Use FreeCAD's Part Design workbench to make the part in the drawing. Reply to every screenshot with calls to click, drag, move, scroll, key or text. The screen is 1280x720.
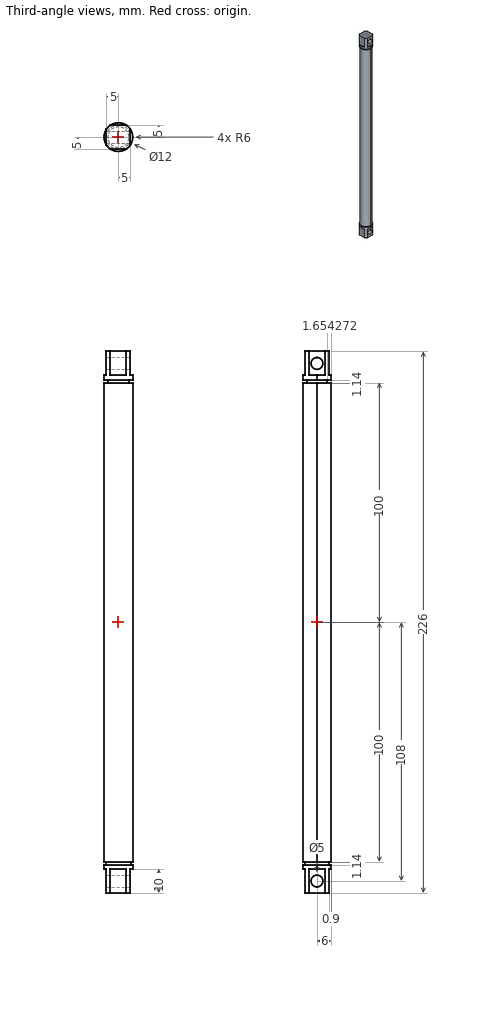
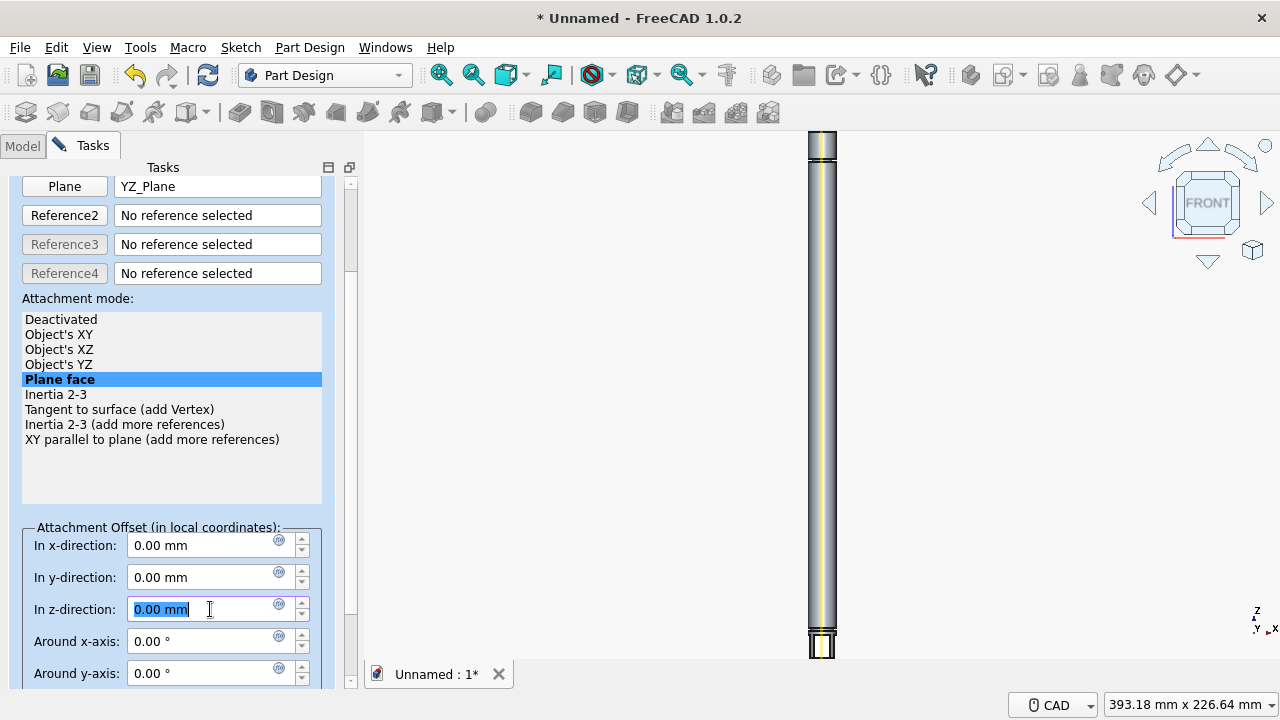
text(-5)
key(Tab)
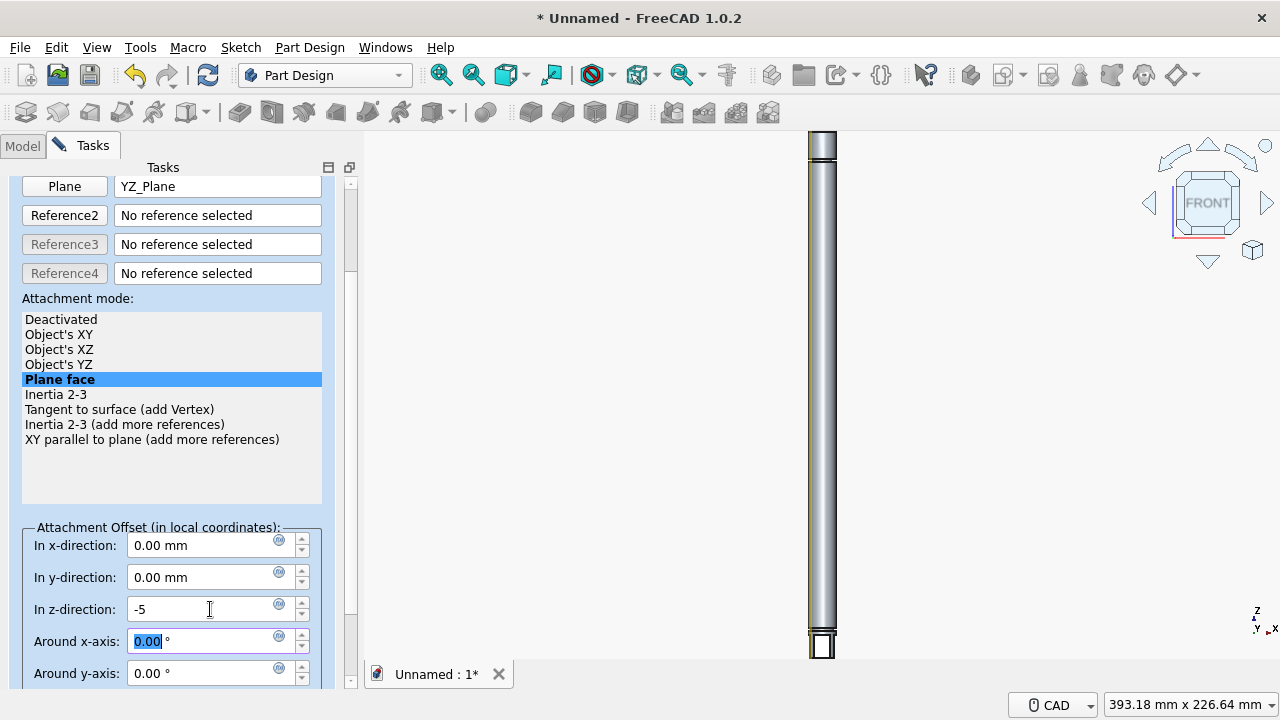
scroll(351, 432, up, 3)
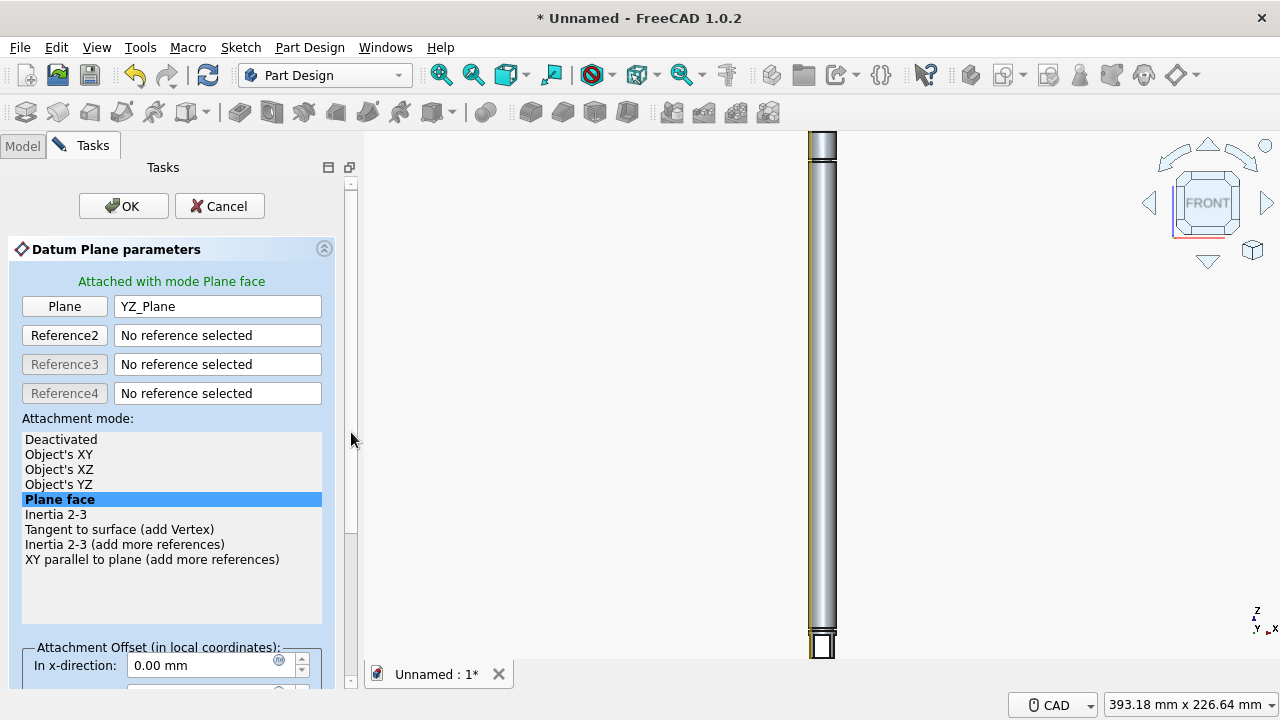
click(124, 206)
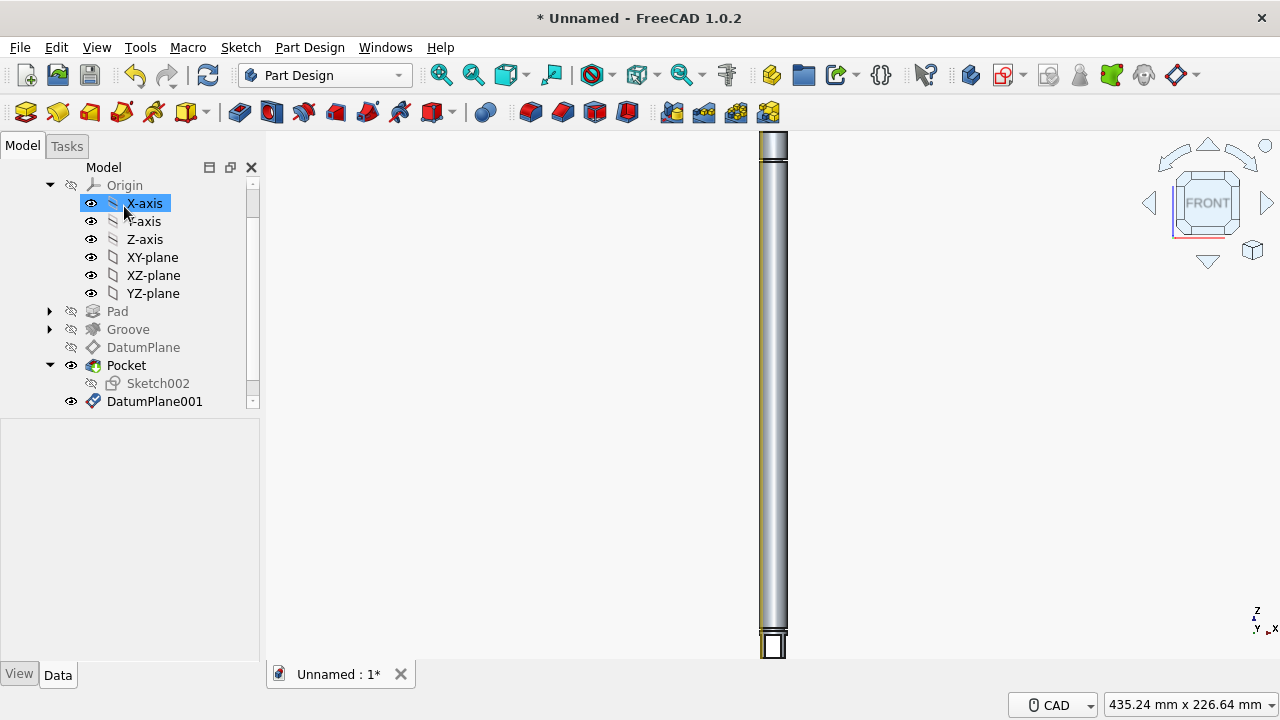
click(116, 401)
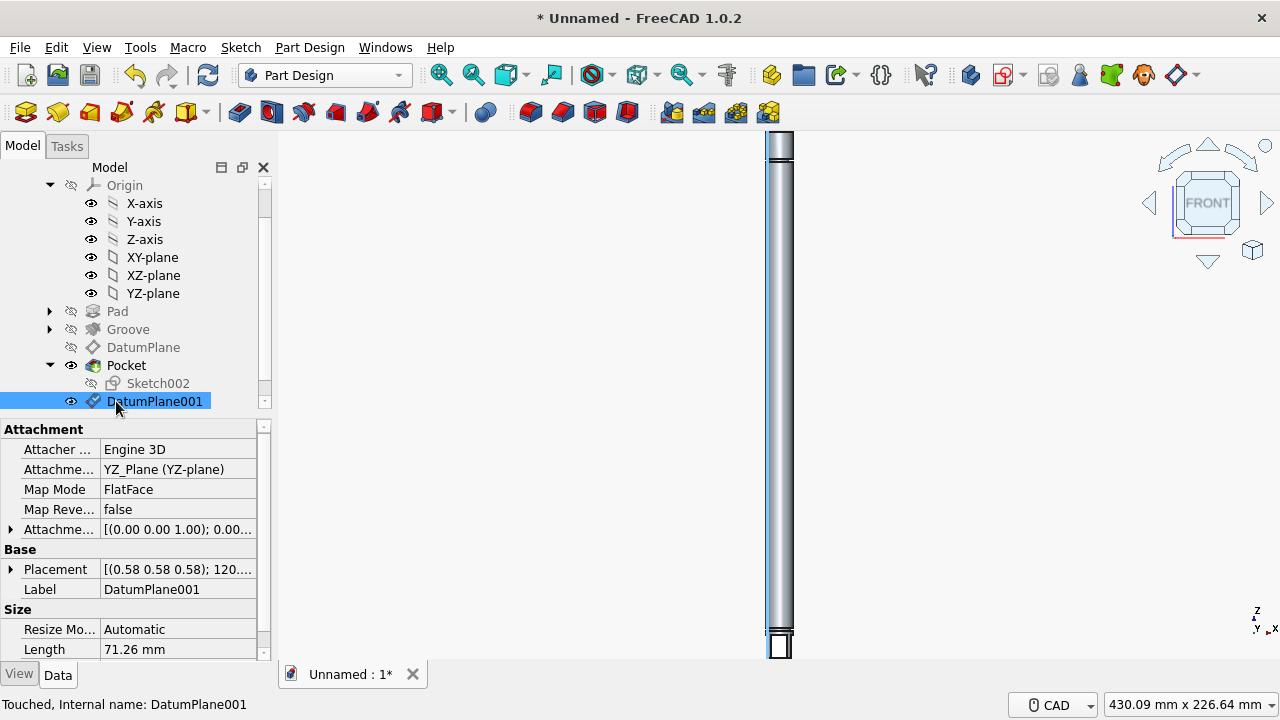
click(1004, 76)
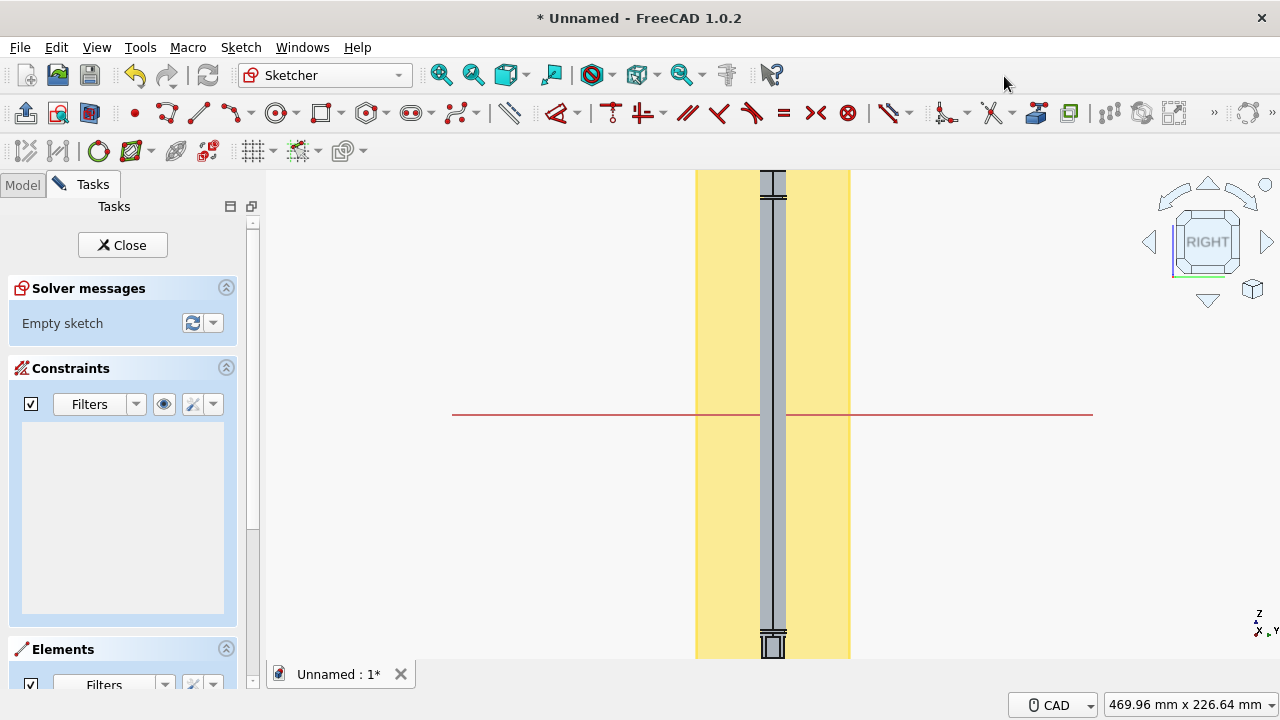
click(90, 114)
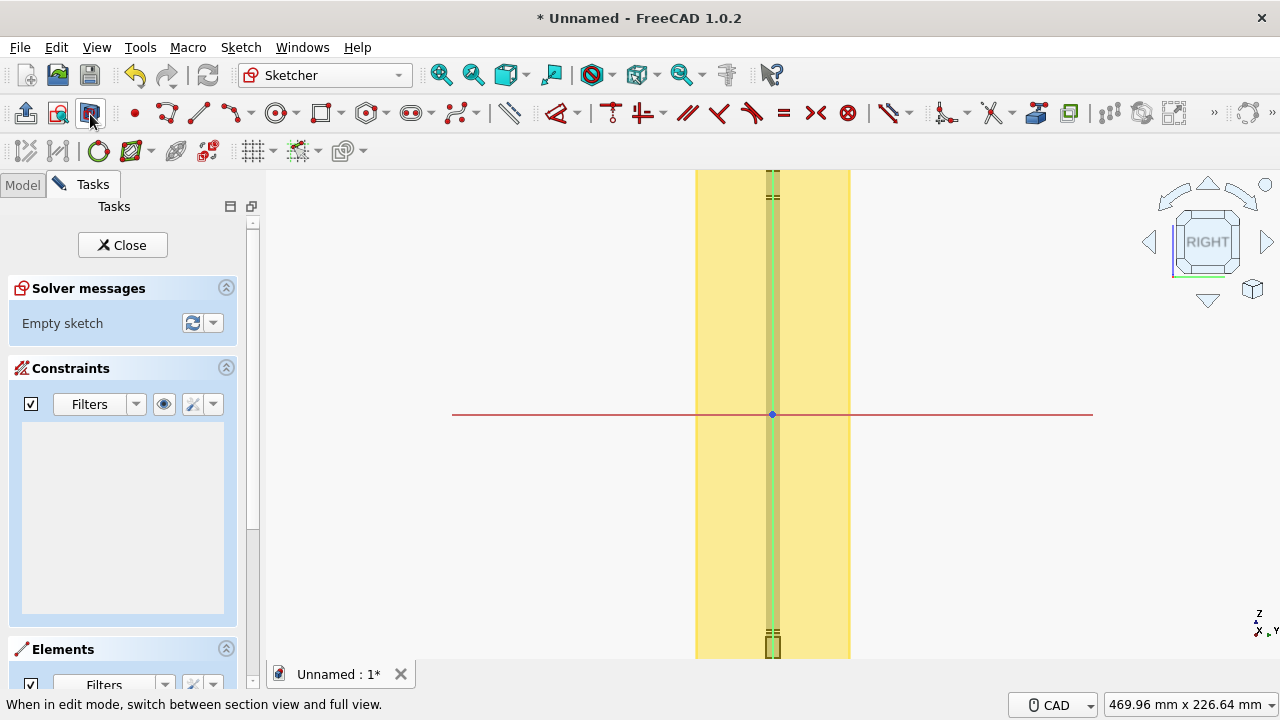
scroll(704, 414, down, 5)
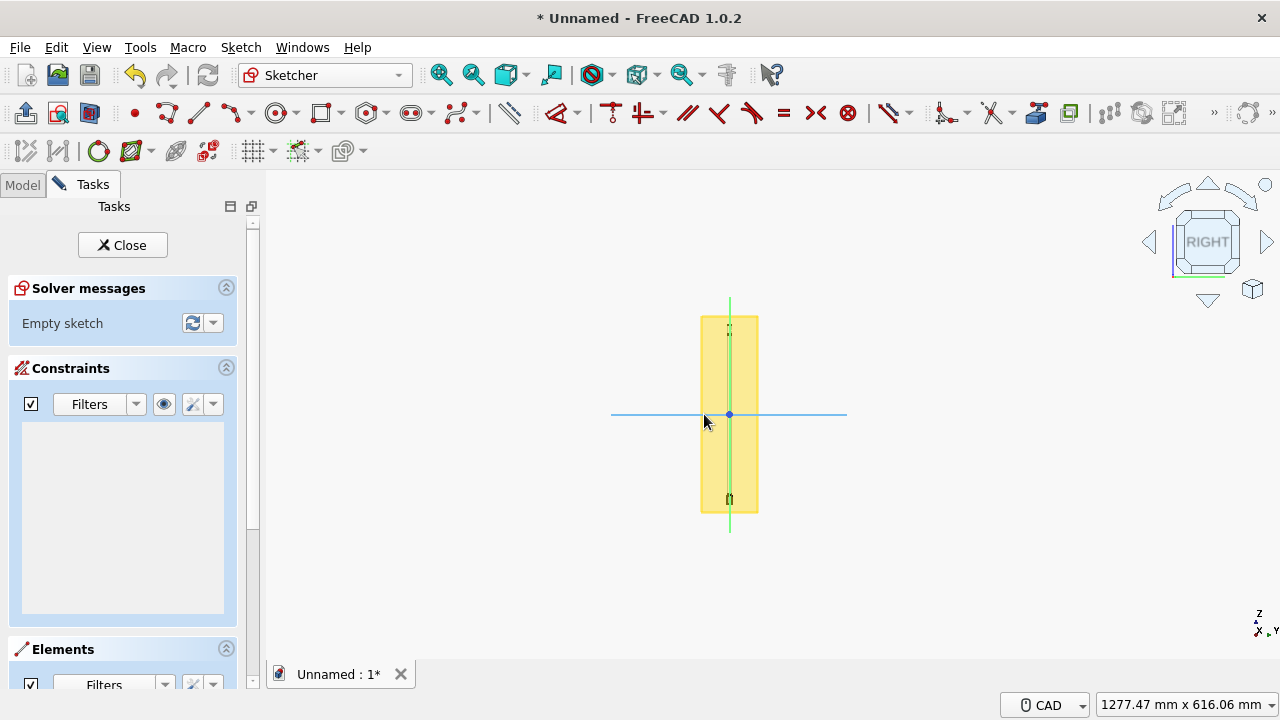
scroll(731, 505, up, 15)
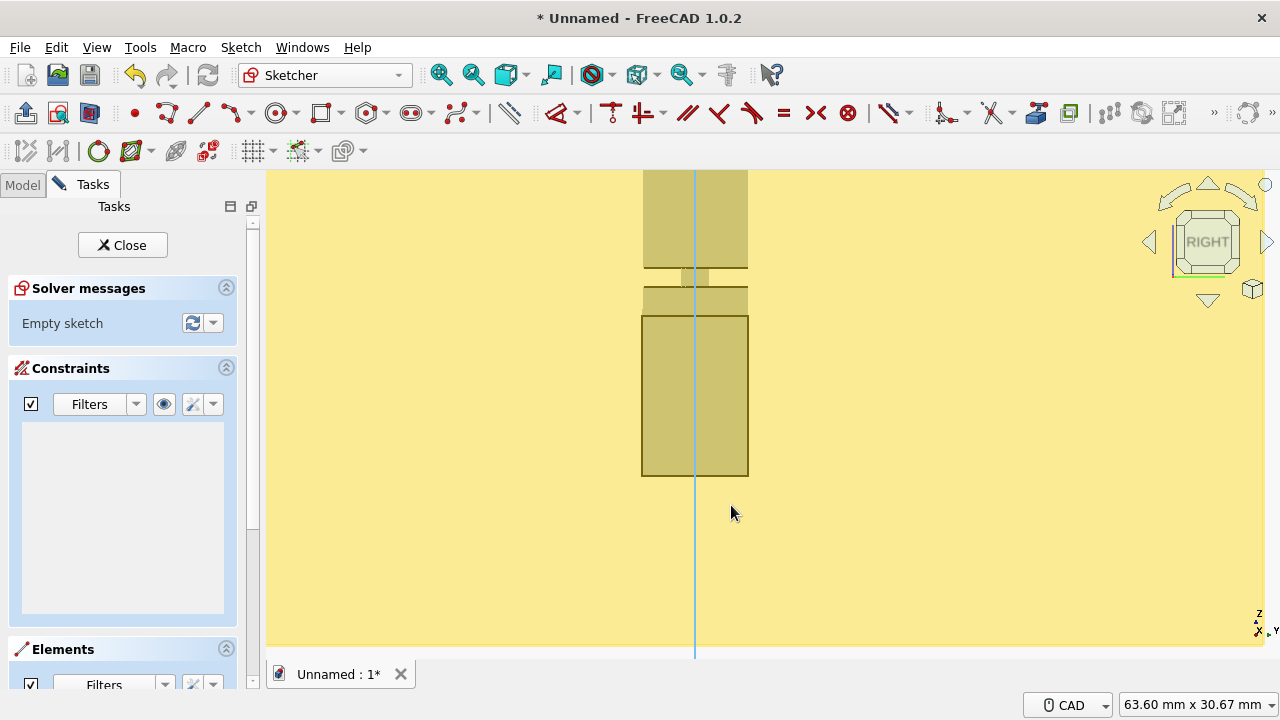
scroll(692, 390, up, 7)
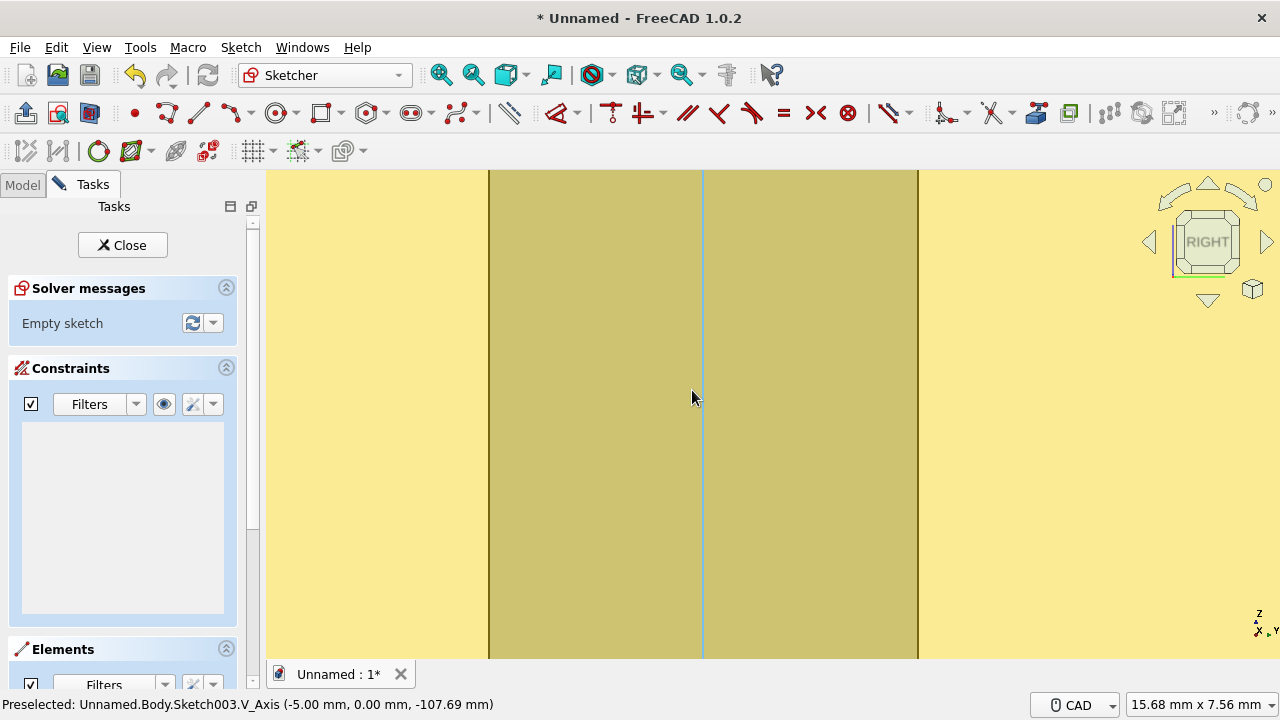
key(g)
key(c)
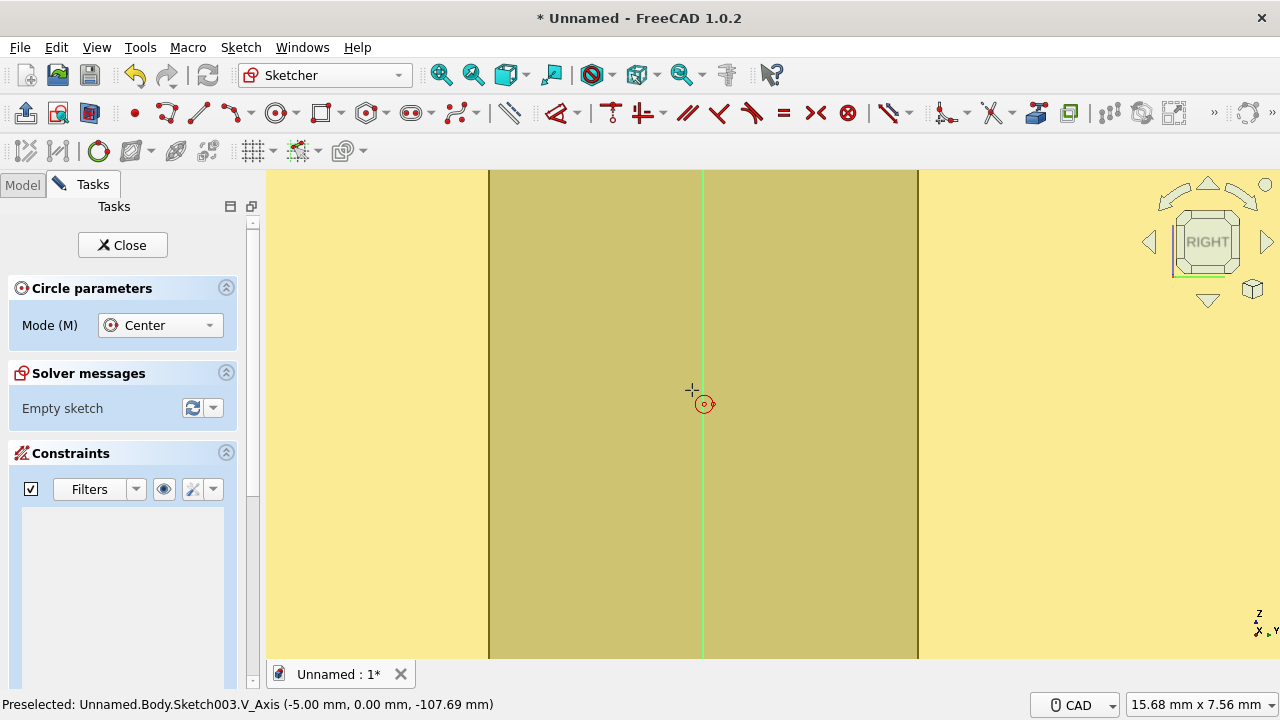
click(703, 413)
move(818, 299)